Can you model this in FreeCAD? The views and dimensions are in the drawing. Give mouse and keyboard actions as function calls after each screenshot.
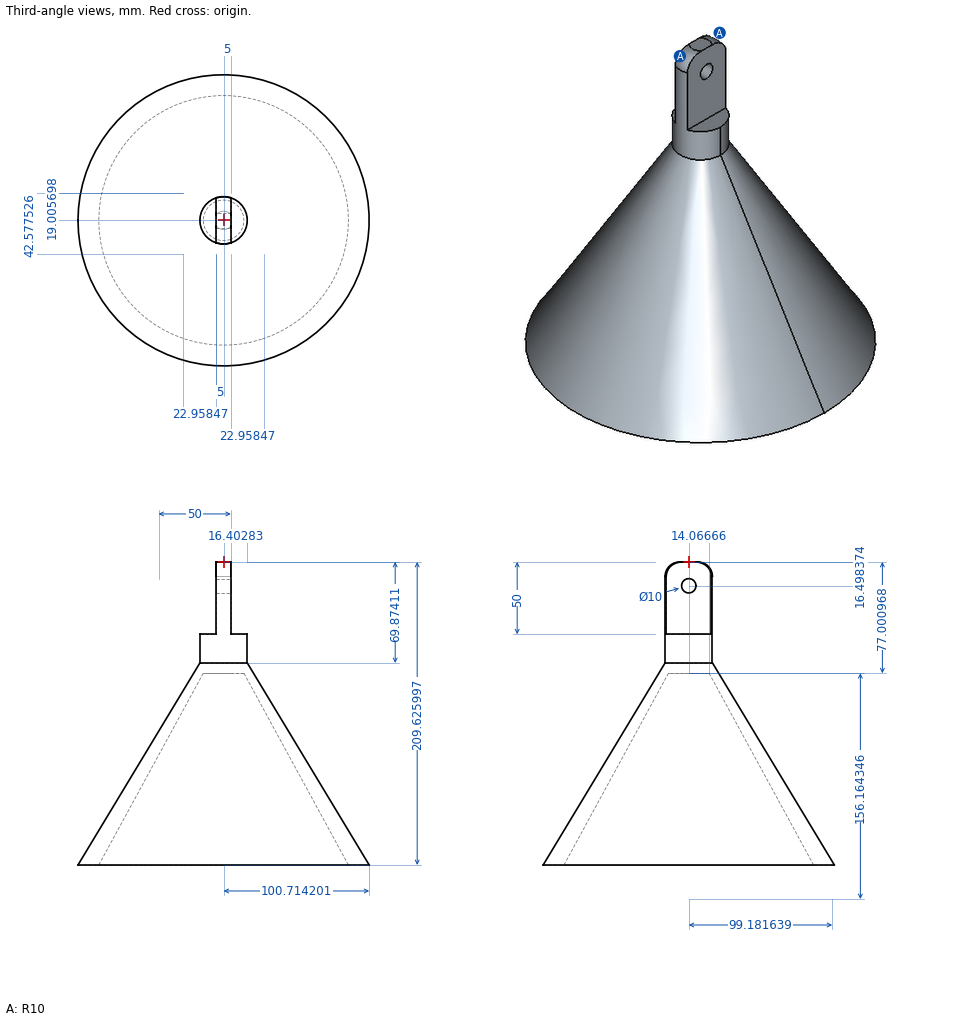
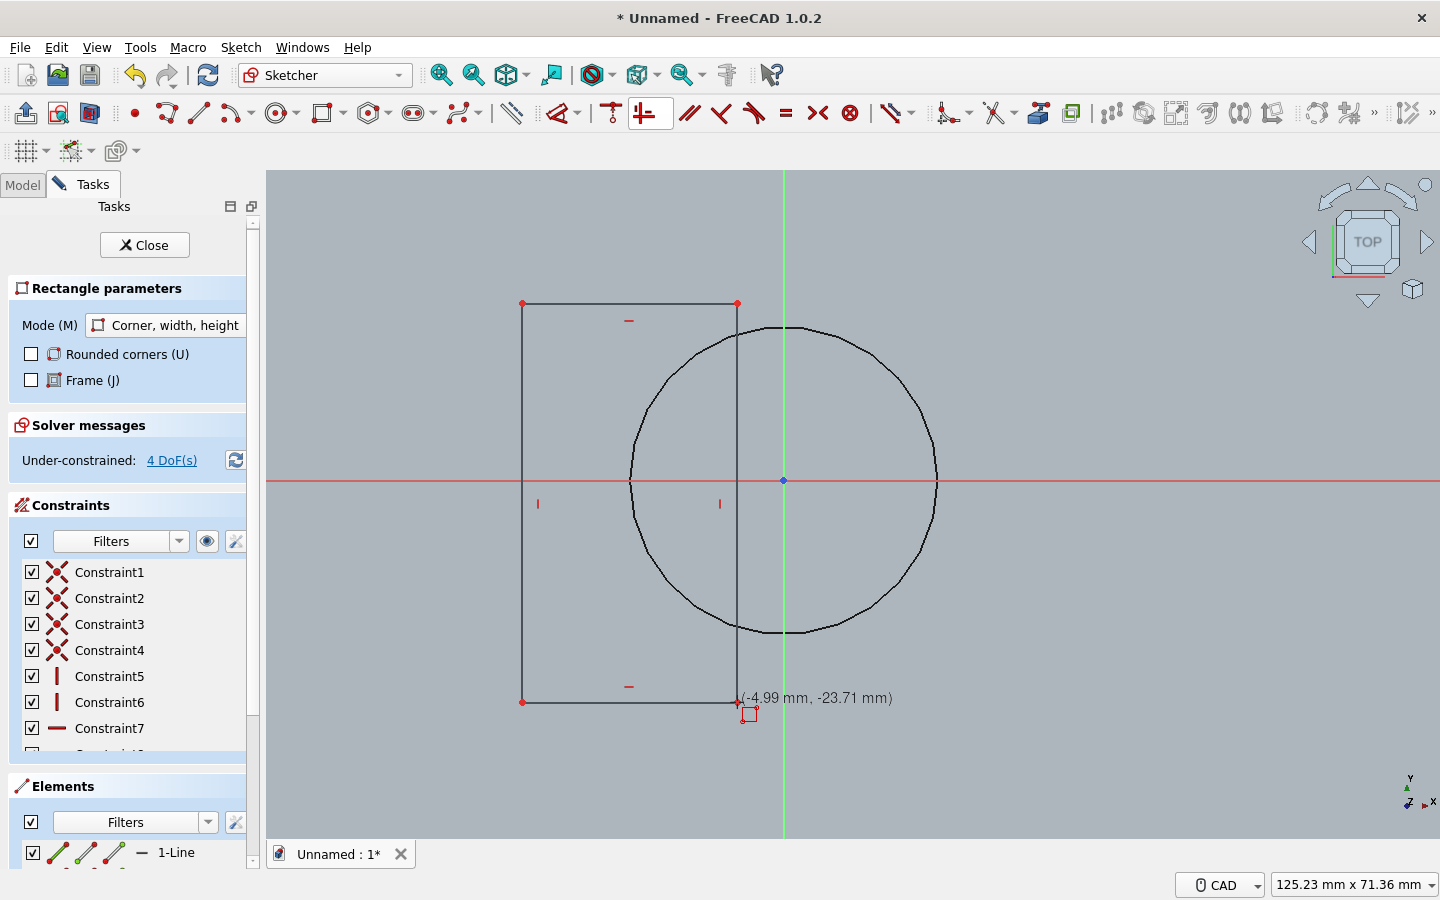
click(831, 303)
click(1046, 702)
key(Escape)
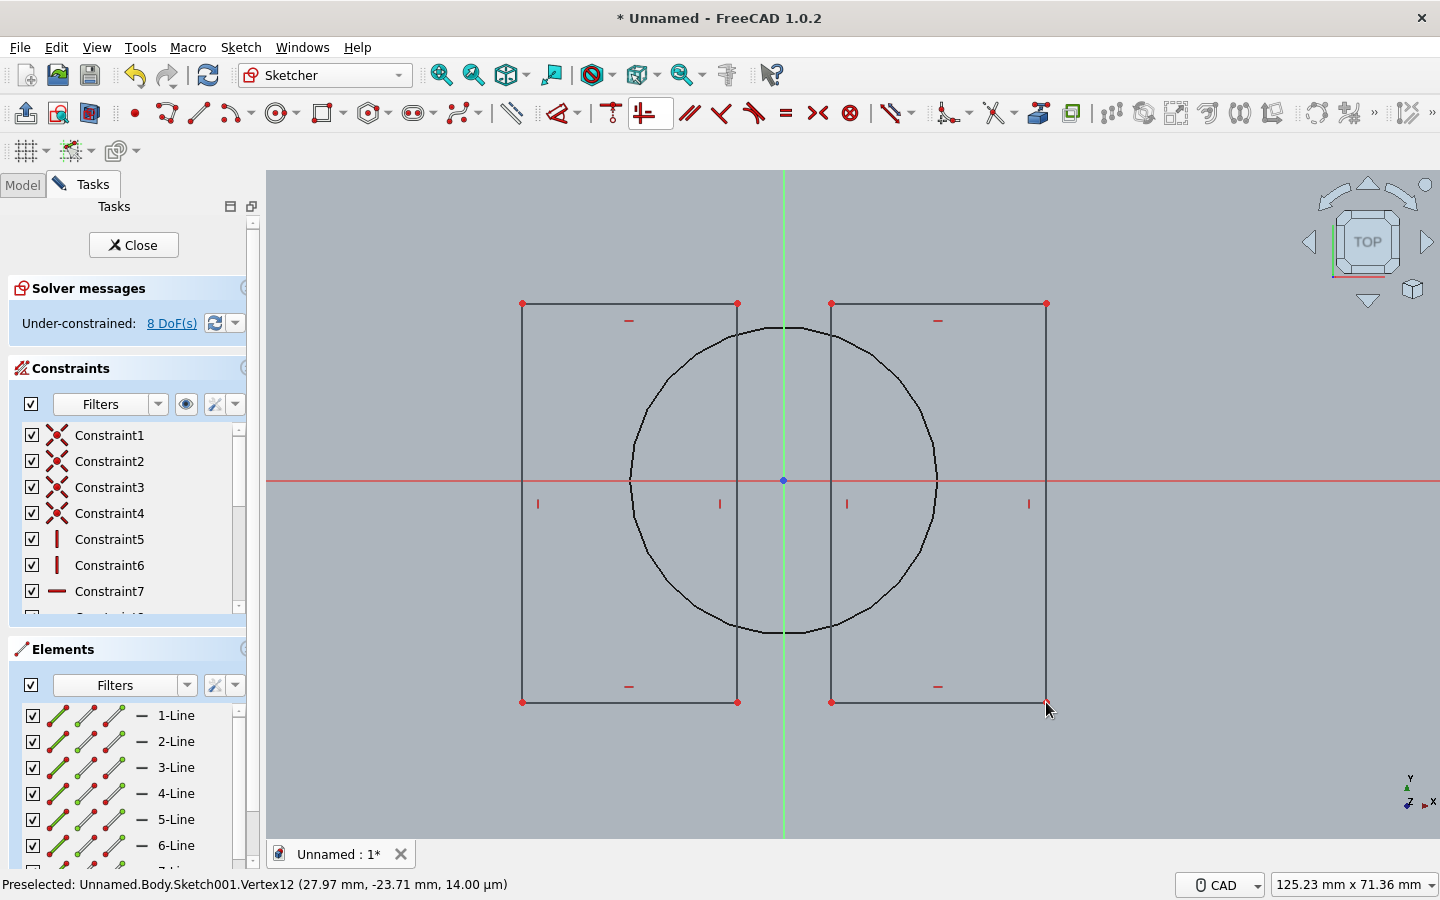
click(558, 114)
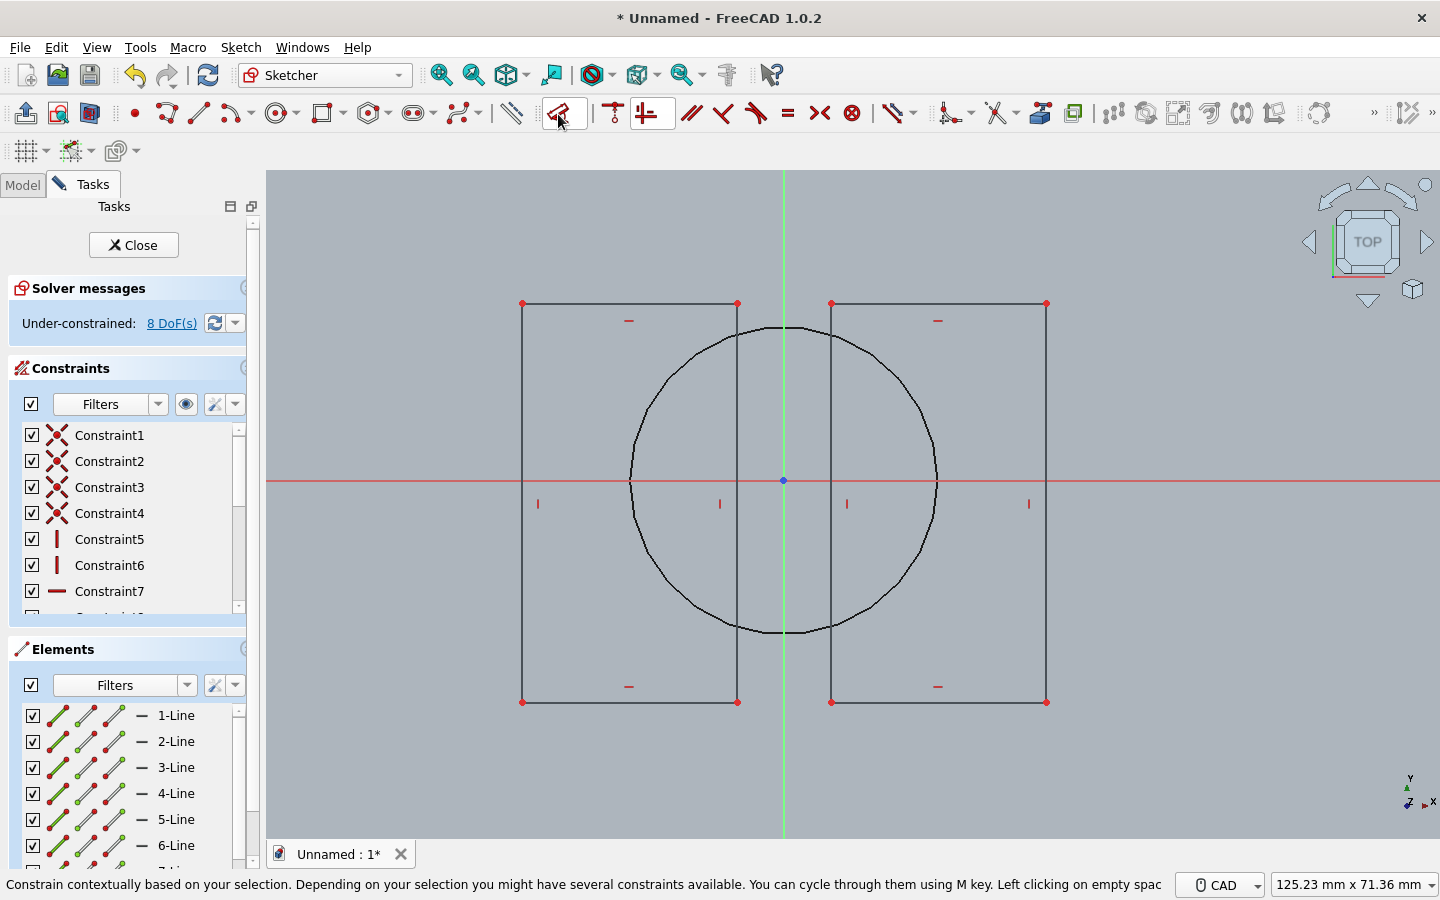
click(737, 703)
click(760, 737)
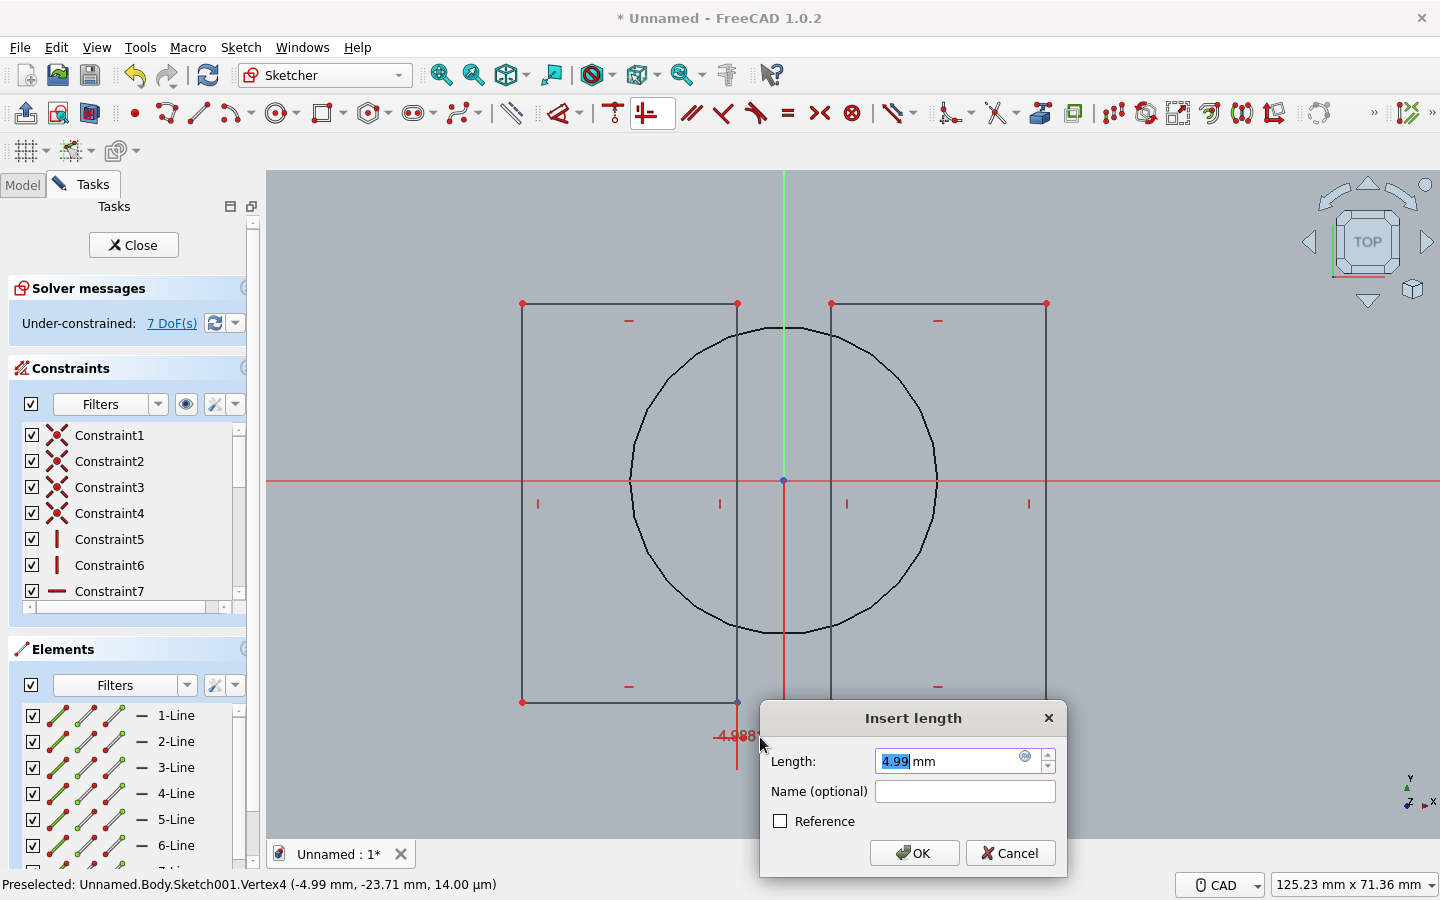
text(5)
key(Return)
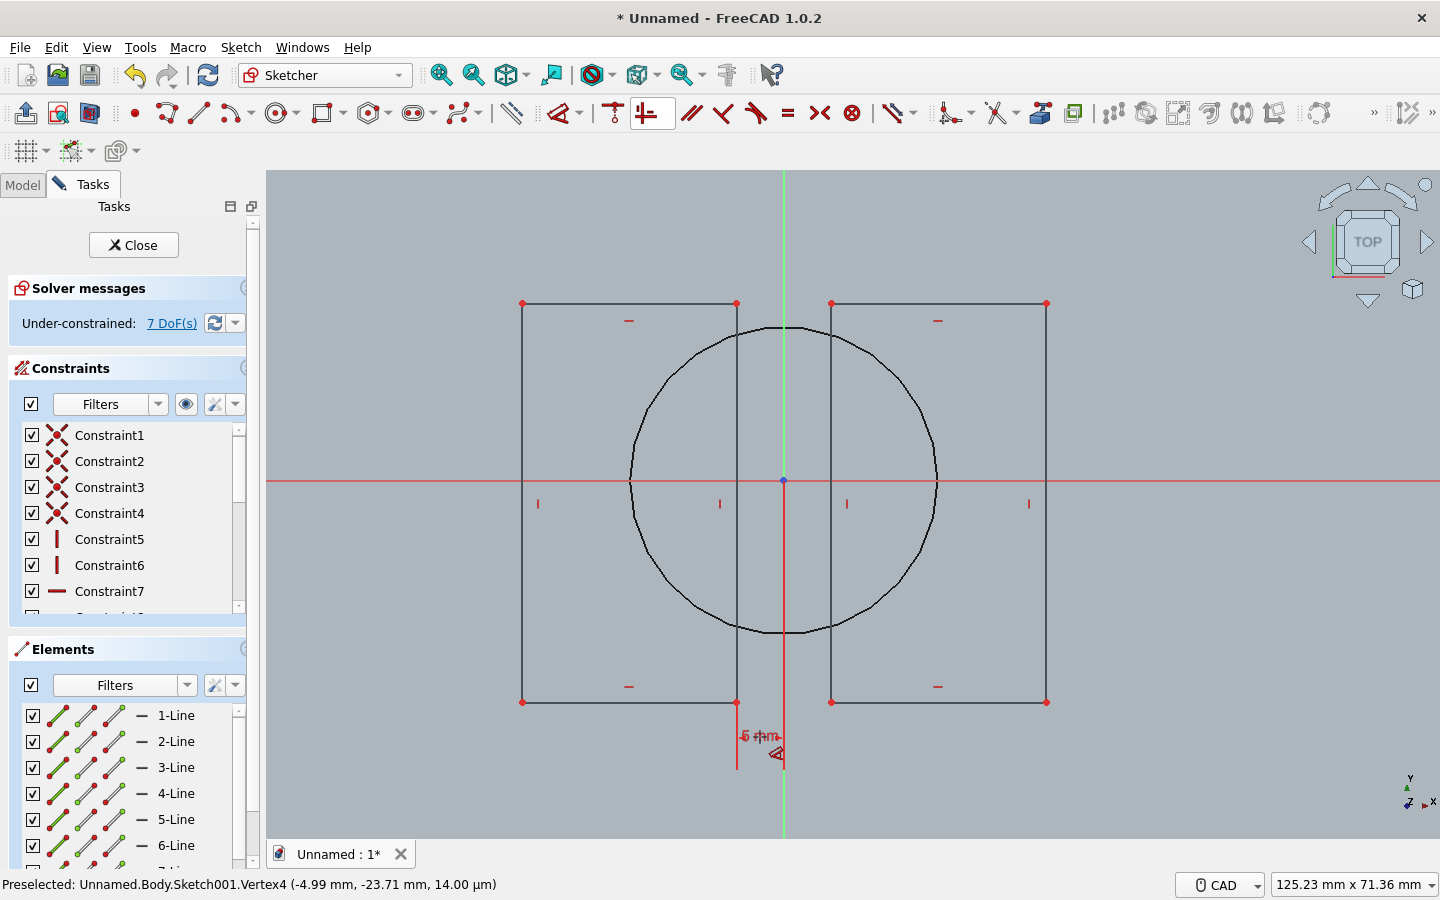
click(831, 304)
click(807, 270)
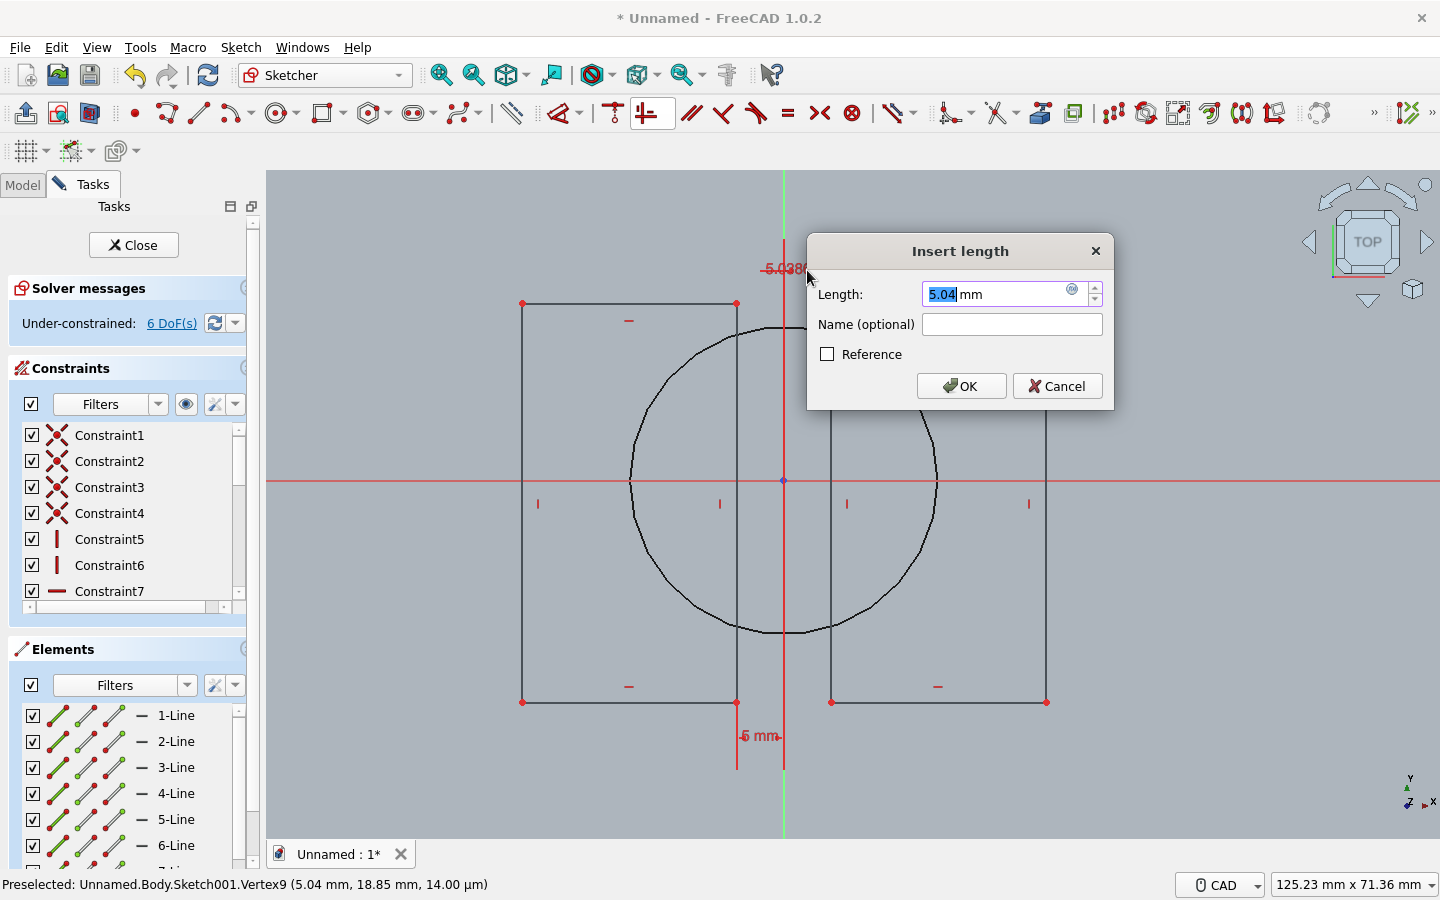
text(5)
key(Return)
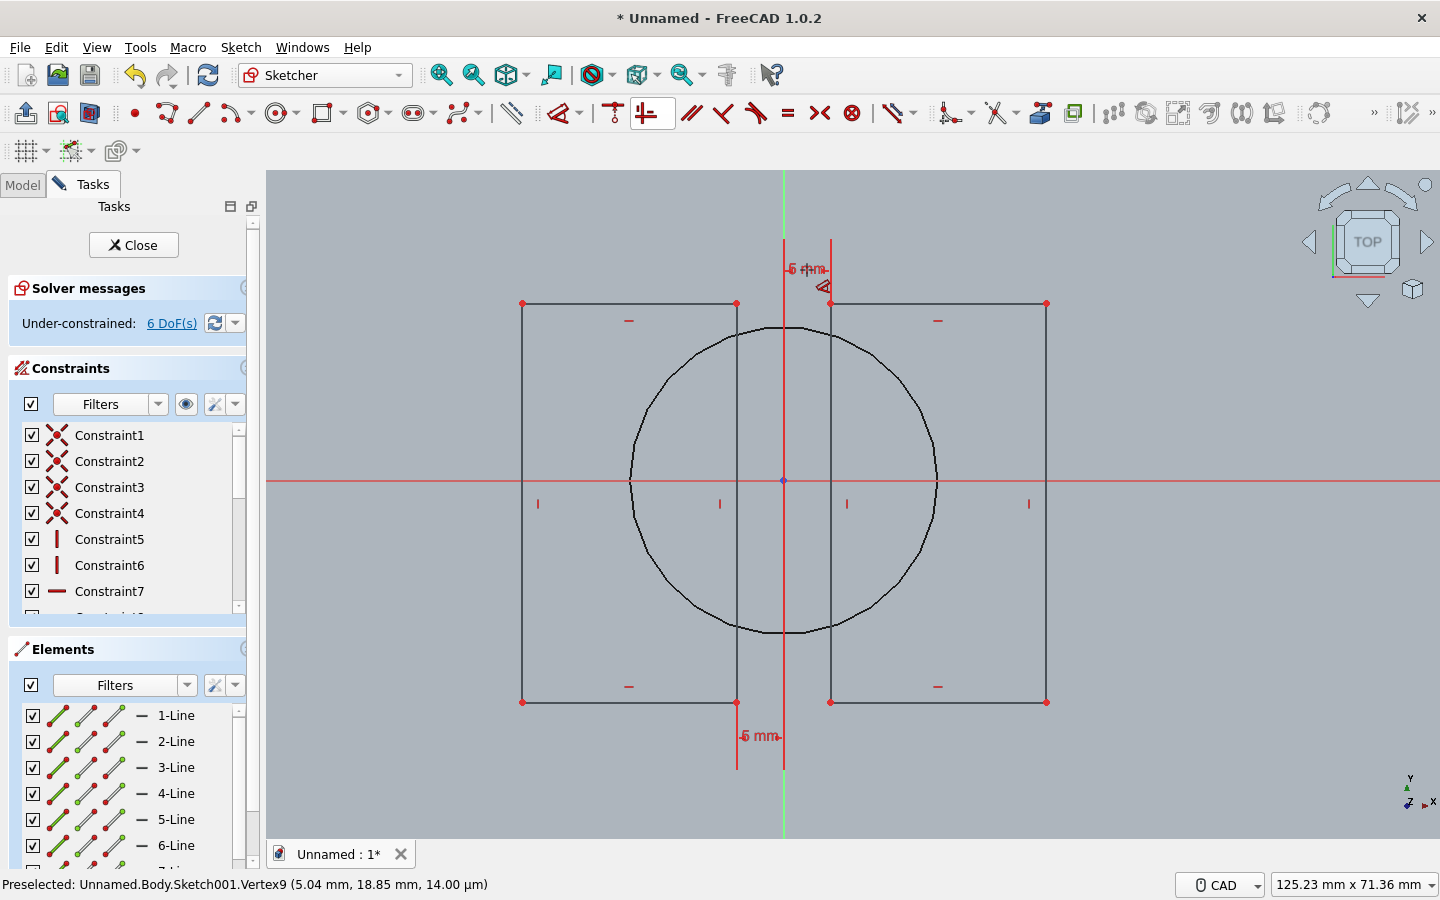
click(586, 703)
click(629, 737)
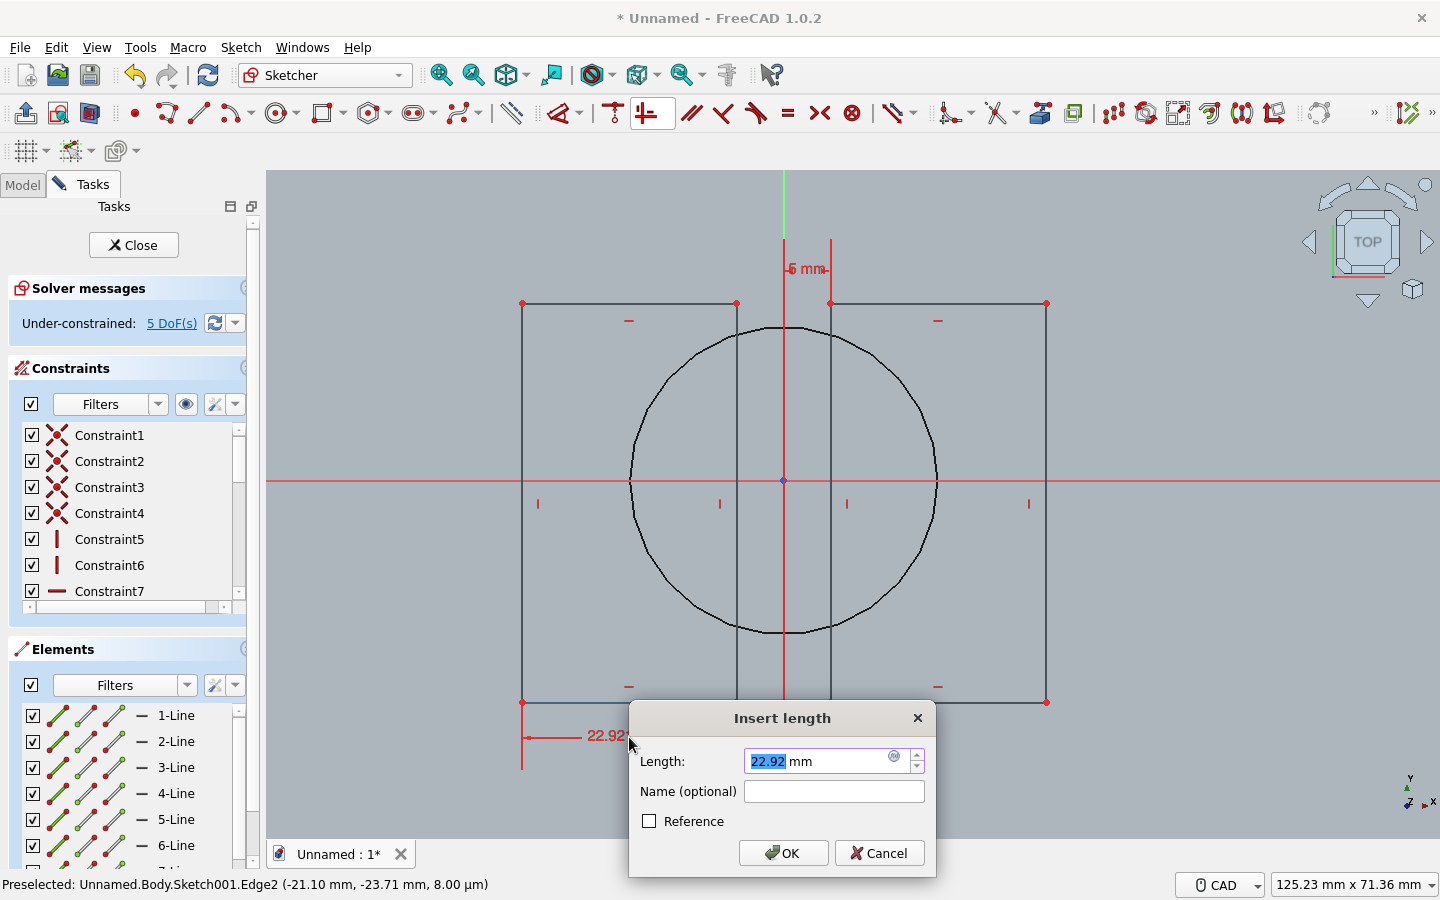
text(22.95847)
key(Return)